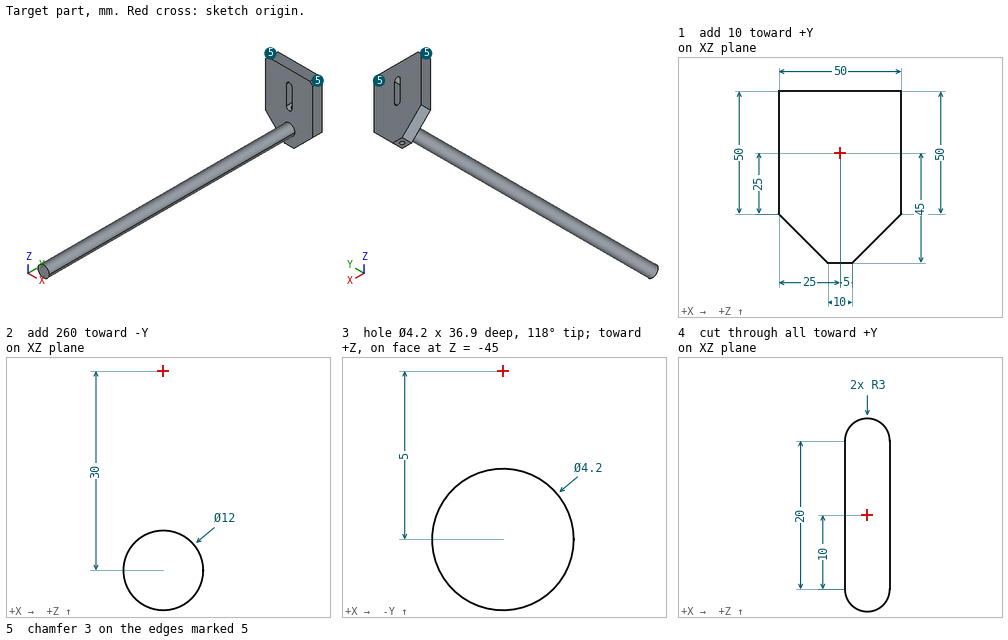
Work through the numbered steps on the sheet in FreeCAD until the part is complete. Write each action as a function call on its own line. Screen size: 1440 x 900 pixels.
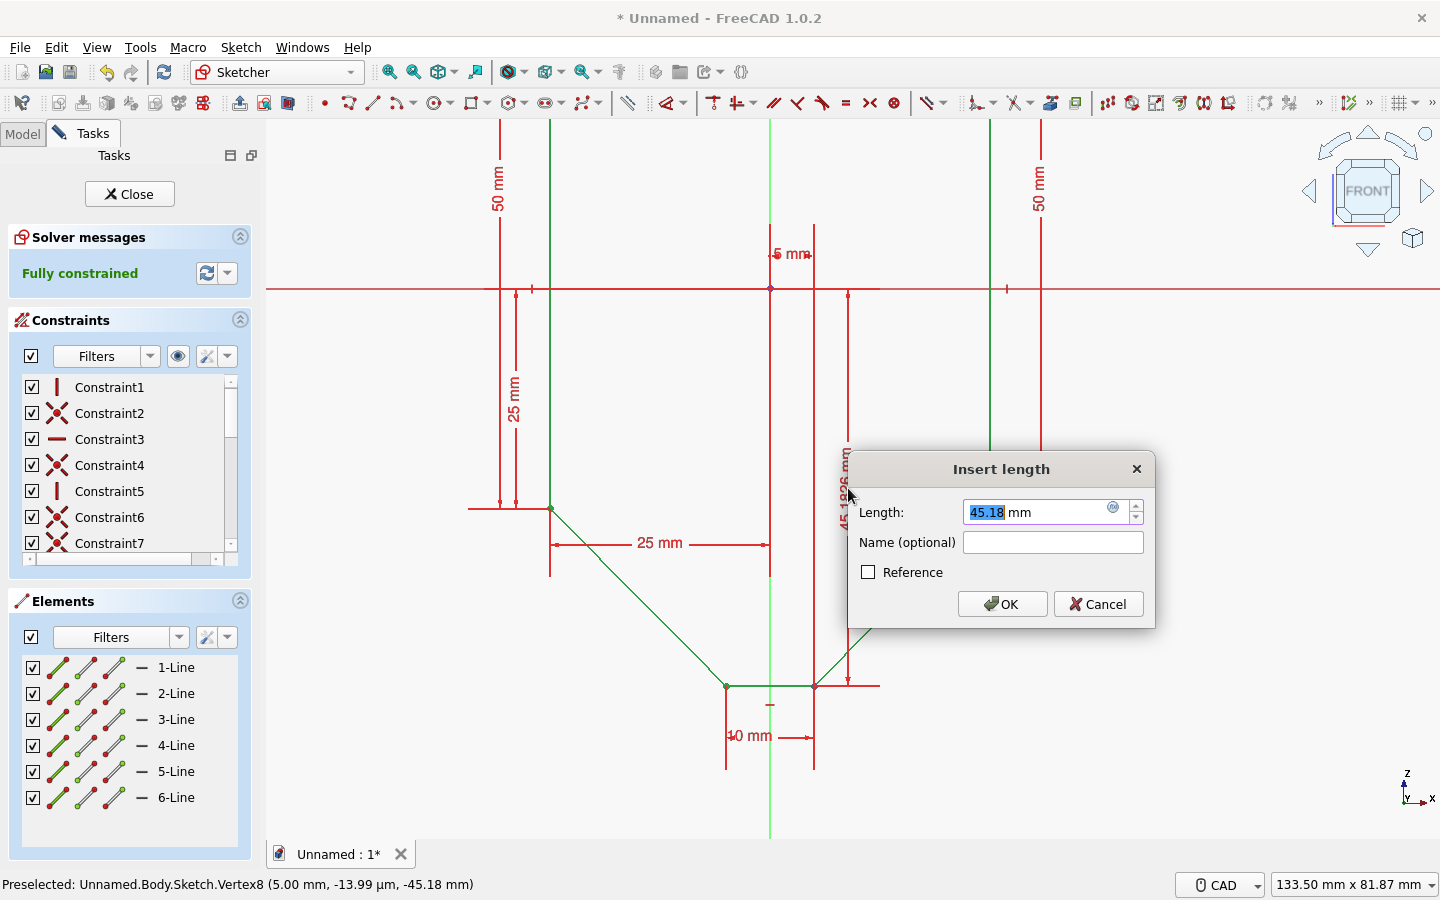
text(45)
key(Return)
key(Escape)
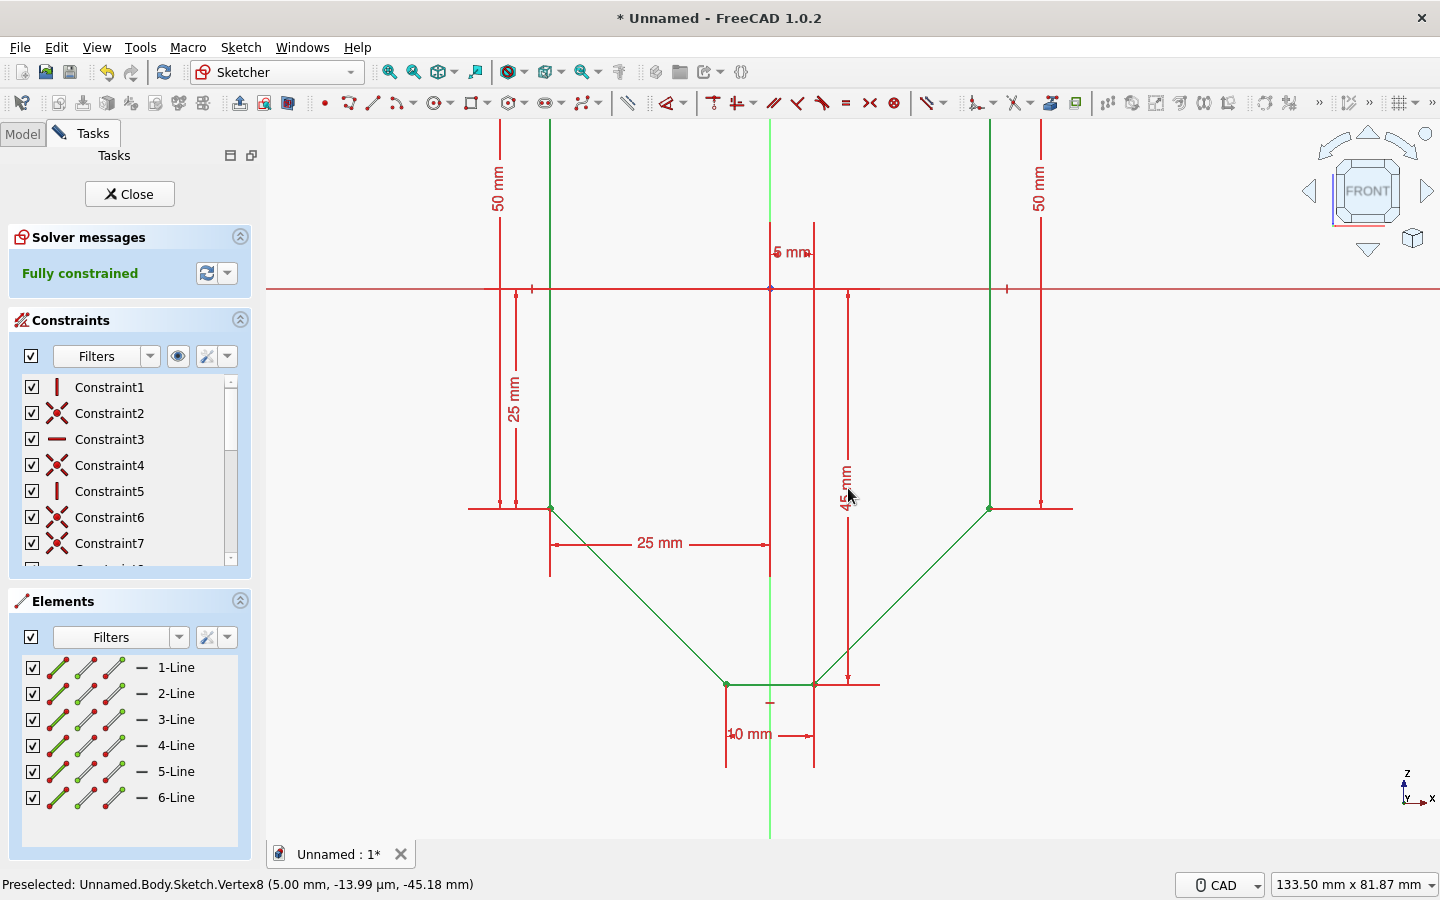
click(130, 194)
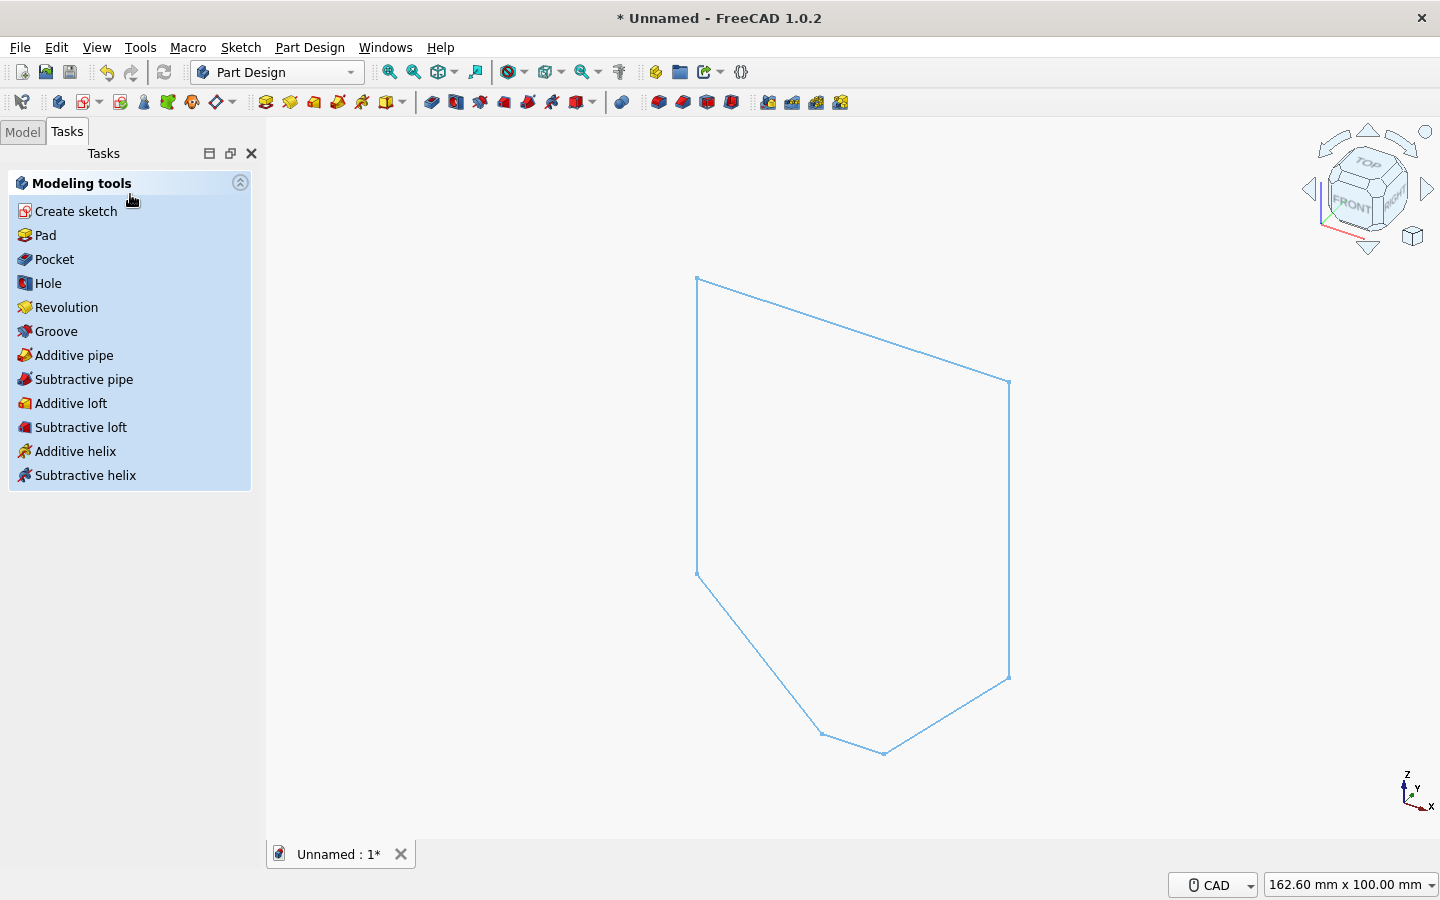
click(266, 102)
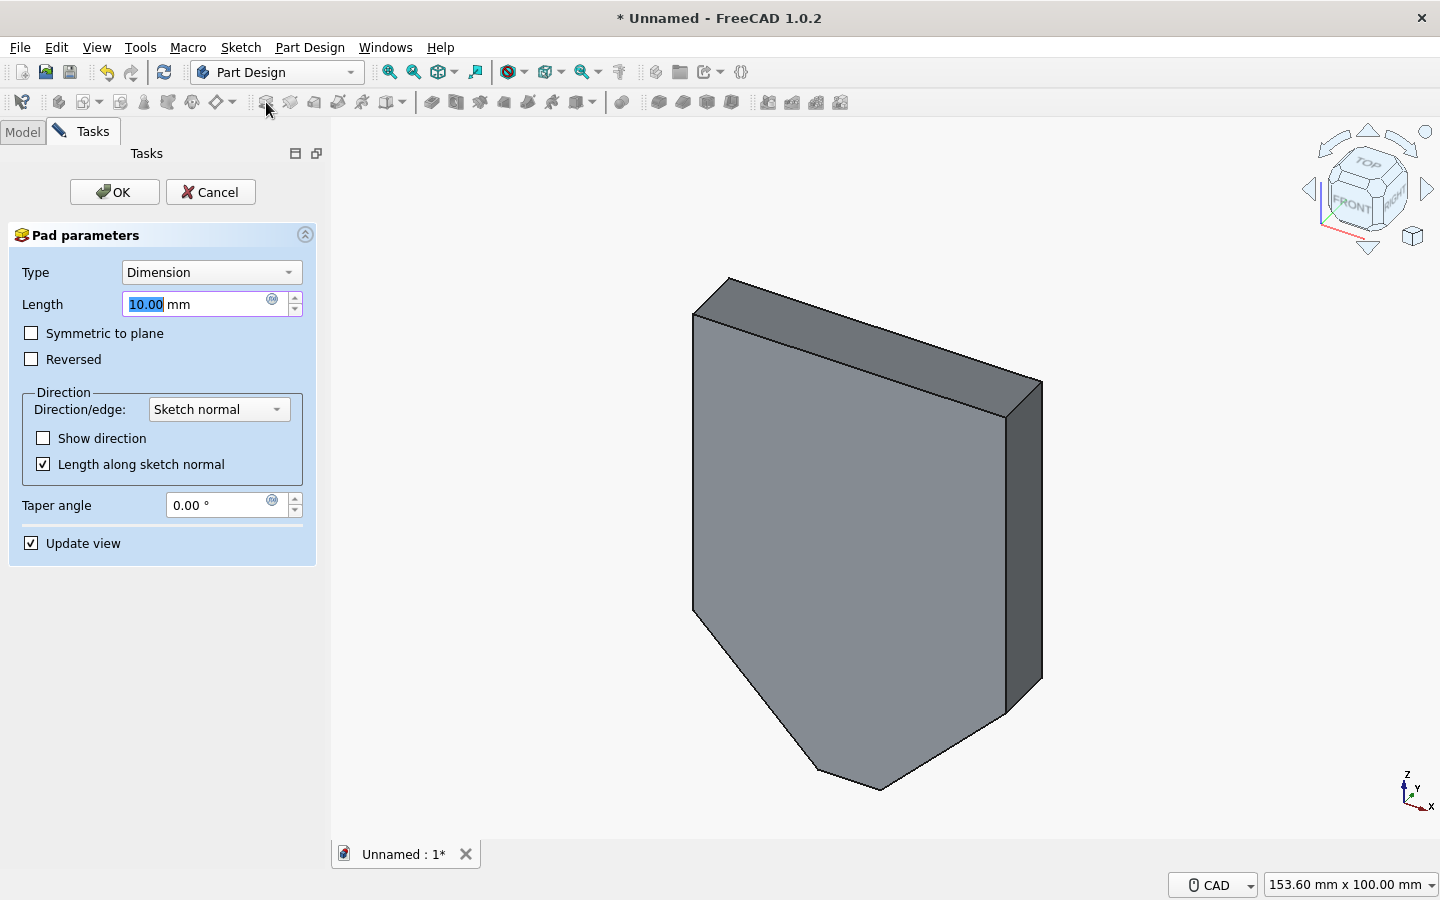
text(10)
key(Tab)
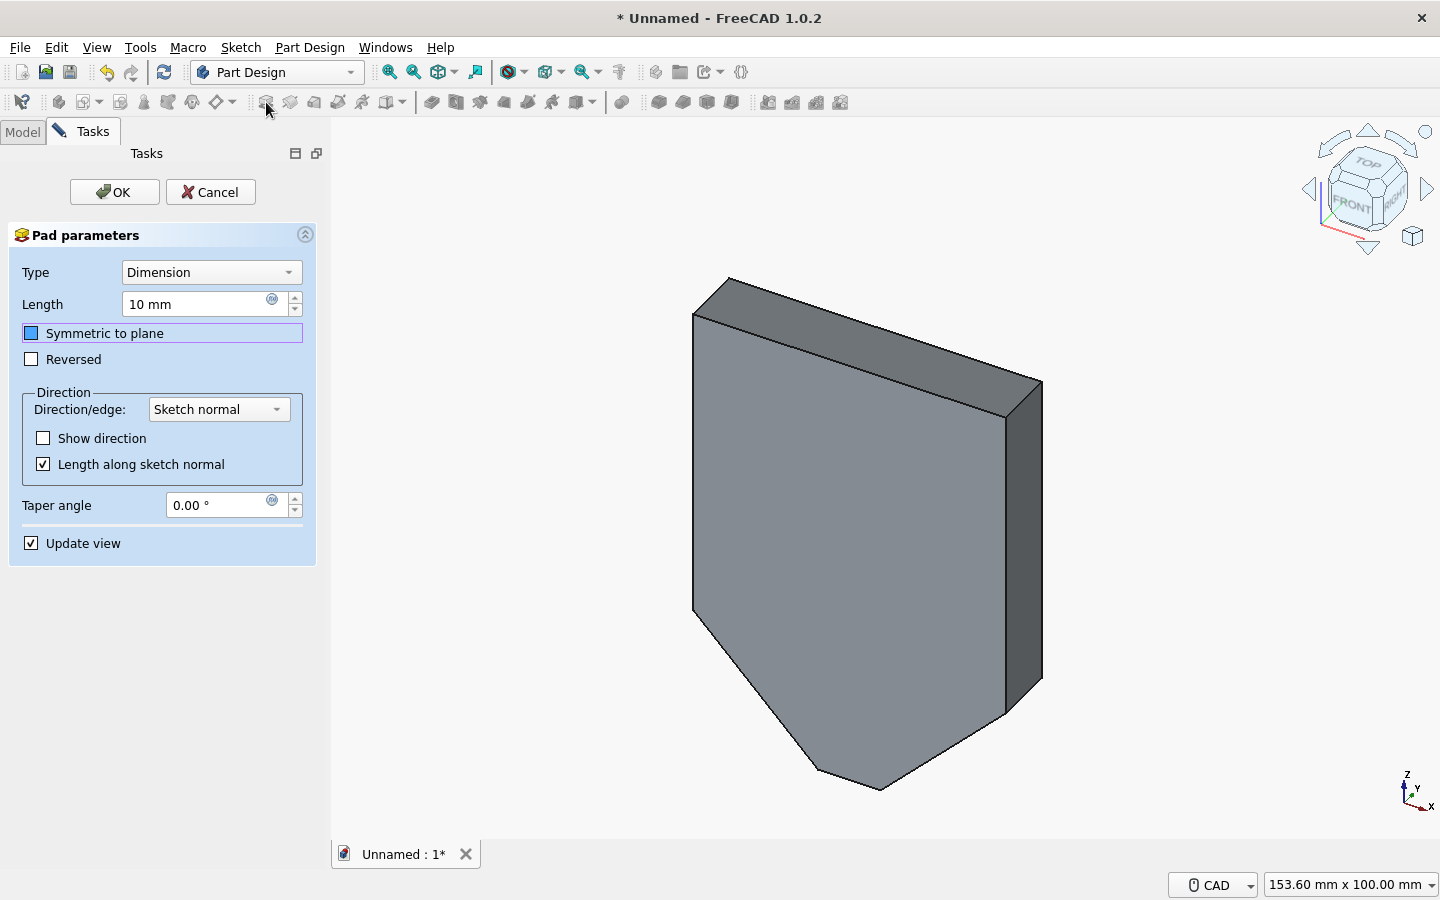
click(30, 359)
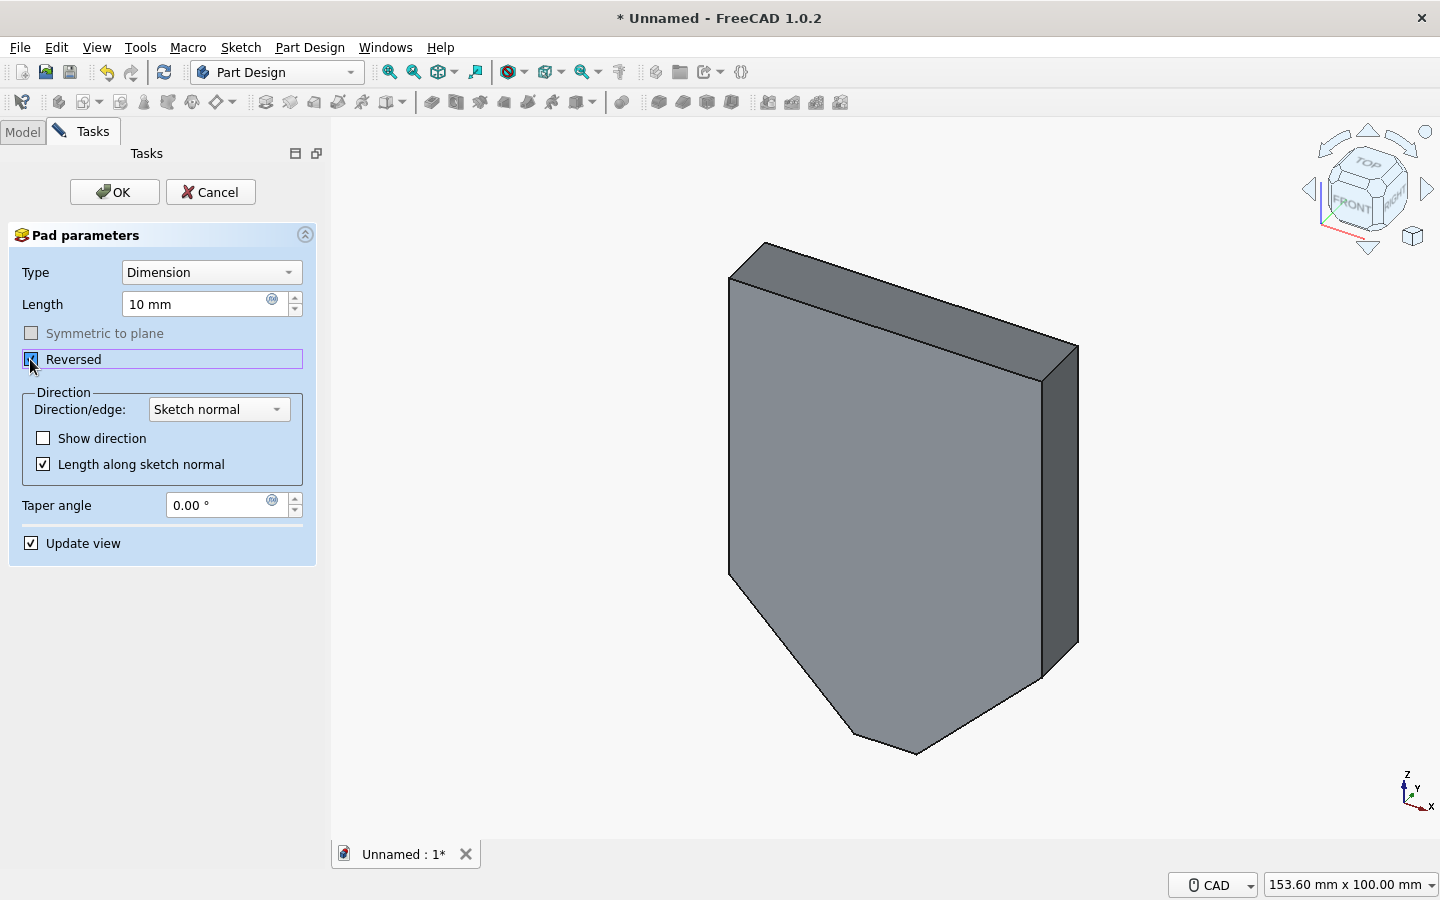
click(115, 192)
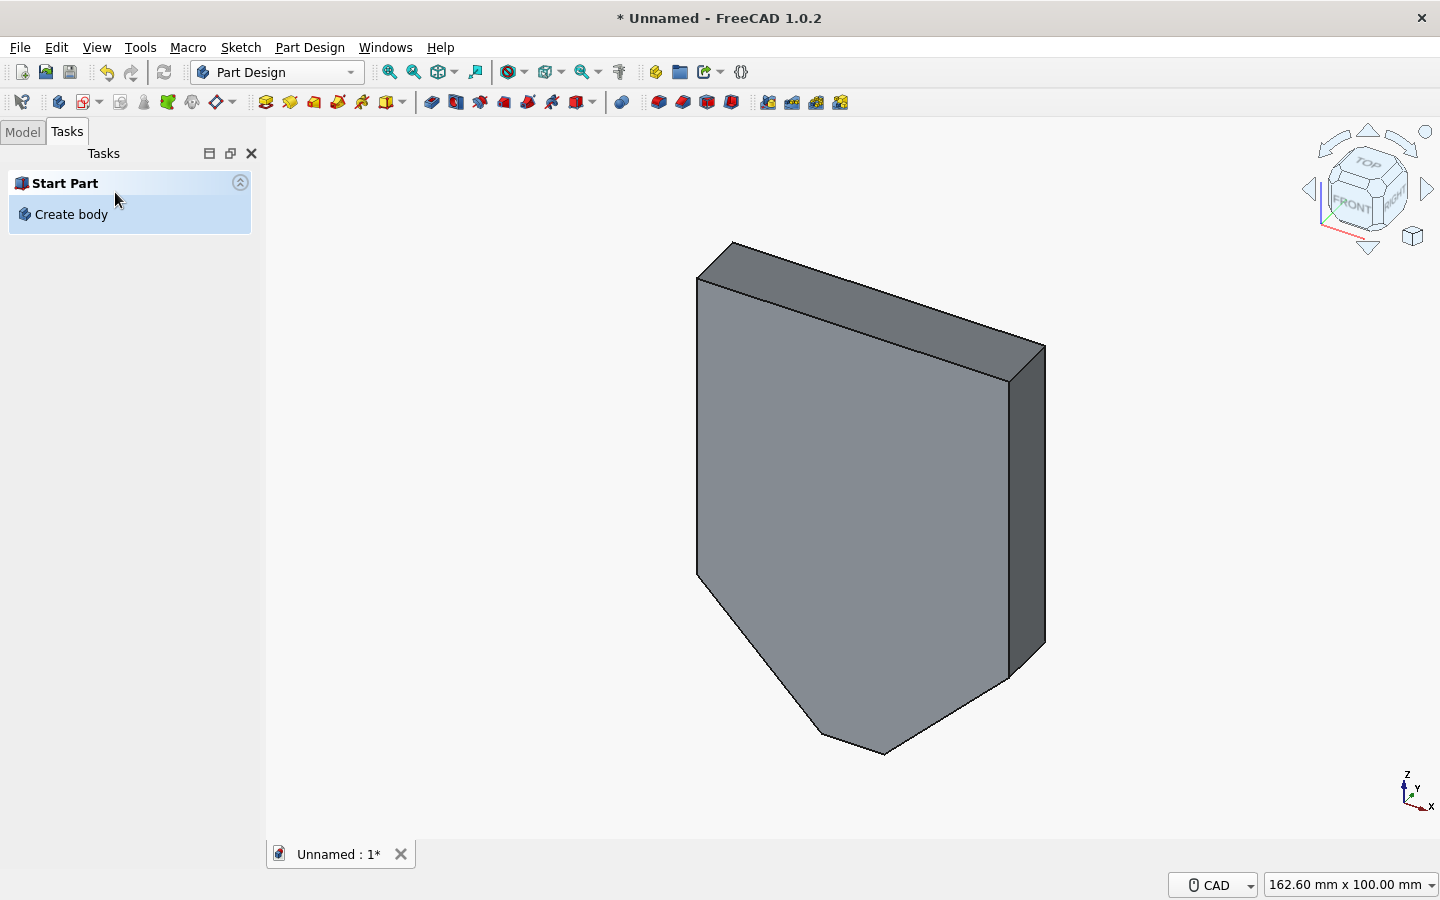
click(84, 102)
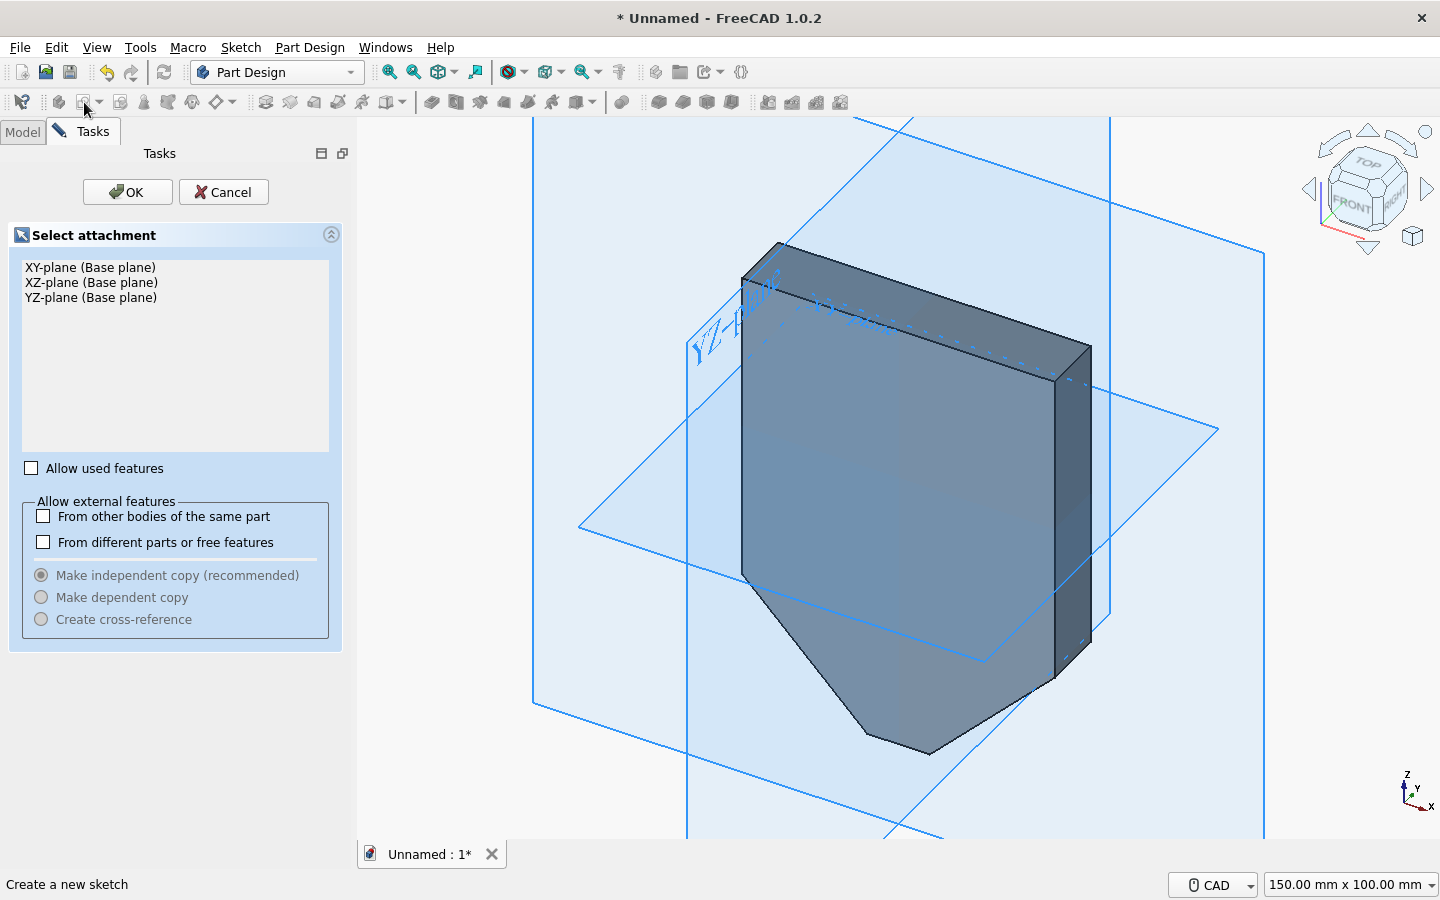
click(82, 282)